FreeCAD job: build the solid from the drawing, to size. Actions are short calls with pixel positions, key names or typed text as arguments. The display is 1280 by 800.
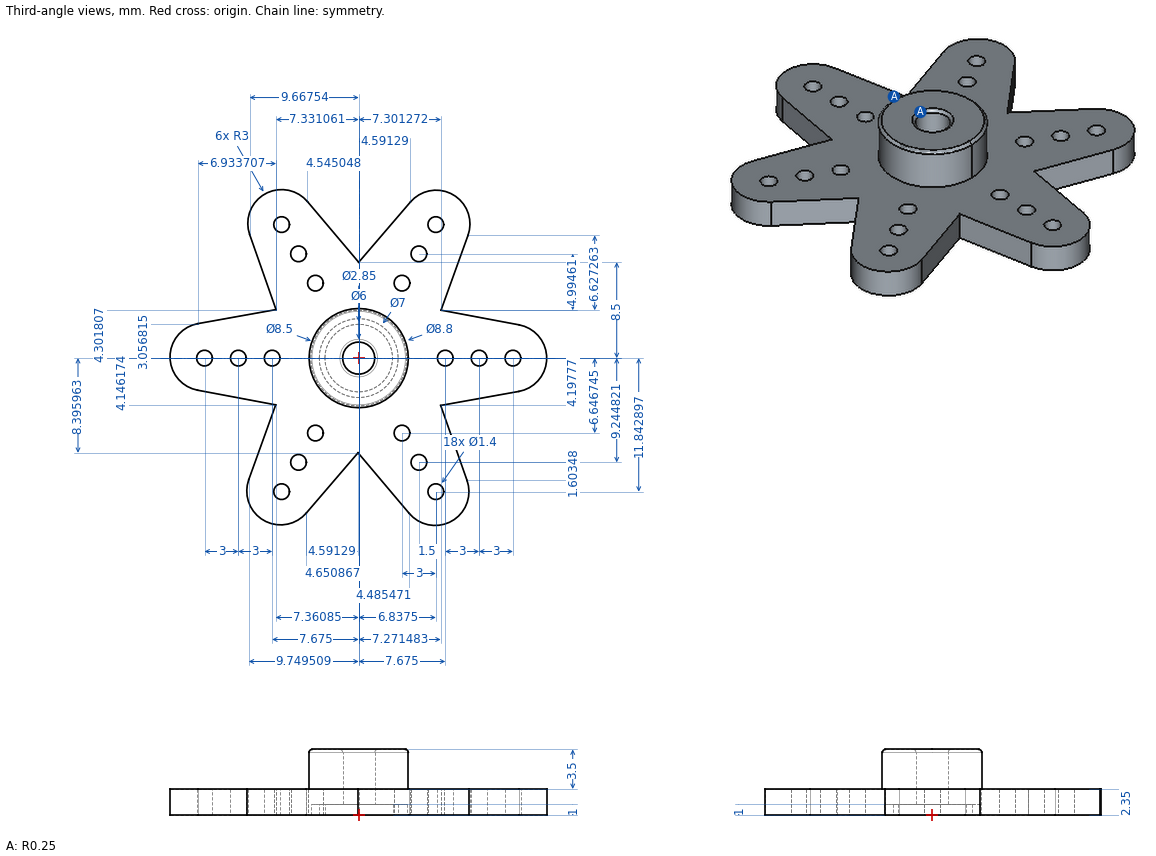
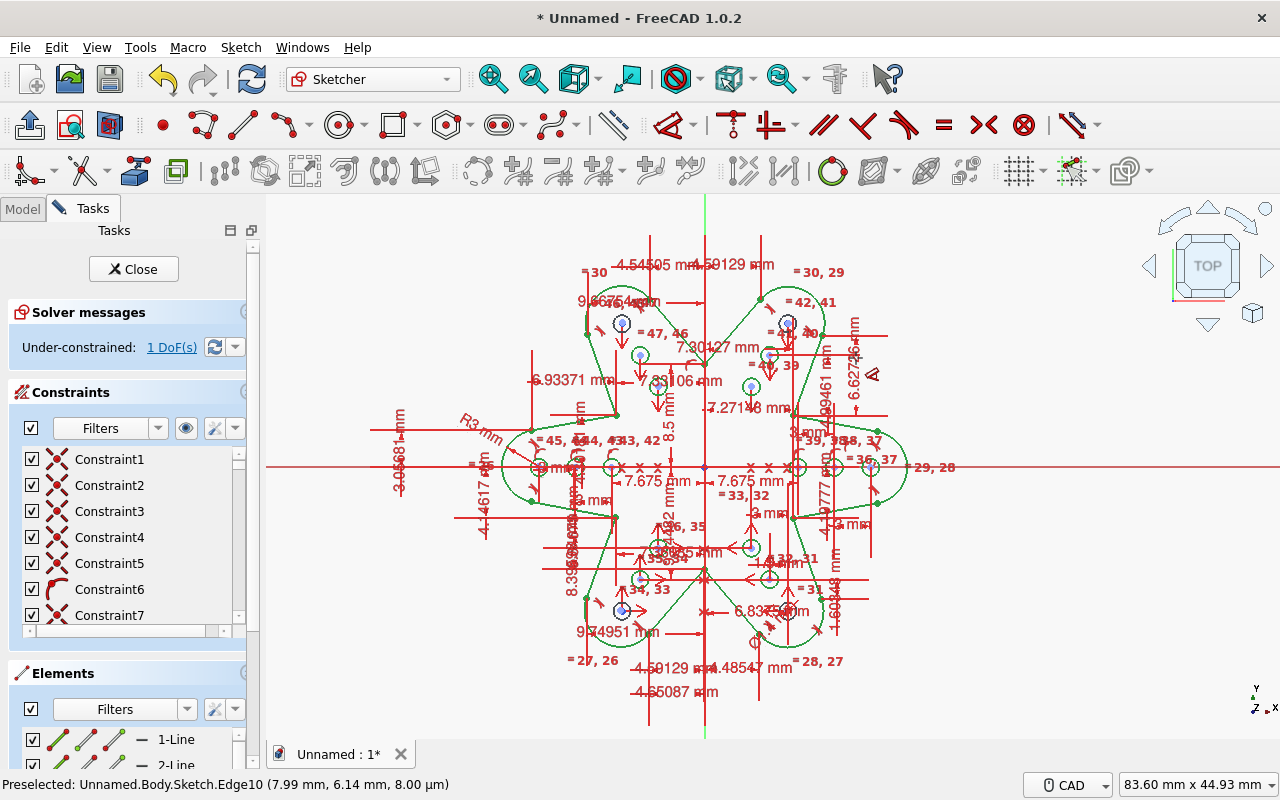
scroll(788, 611, up, 14)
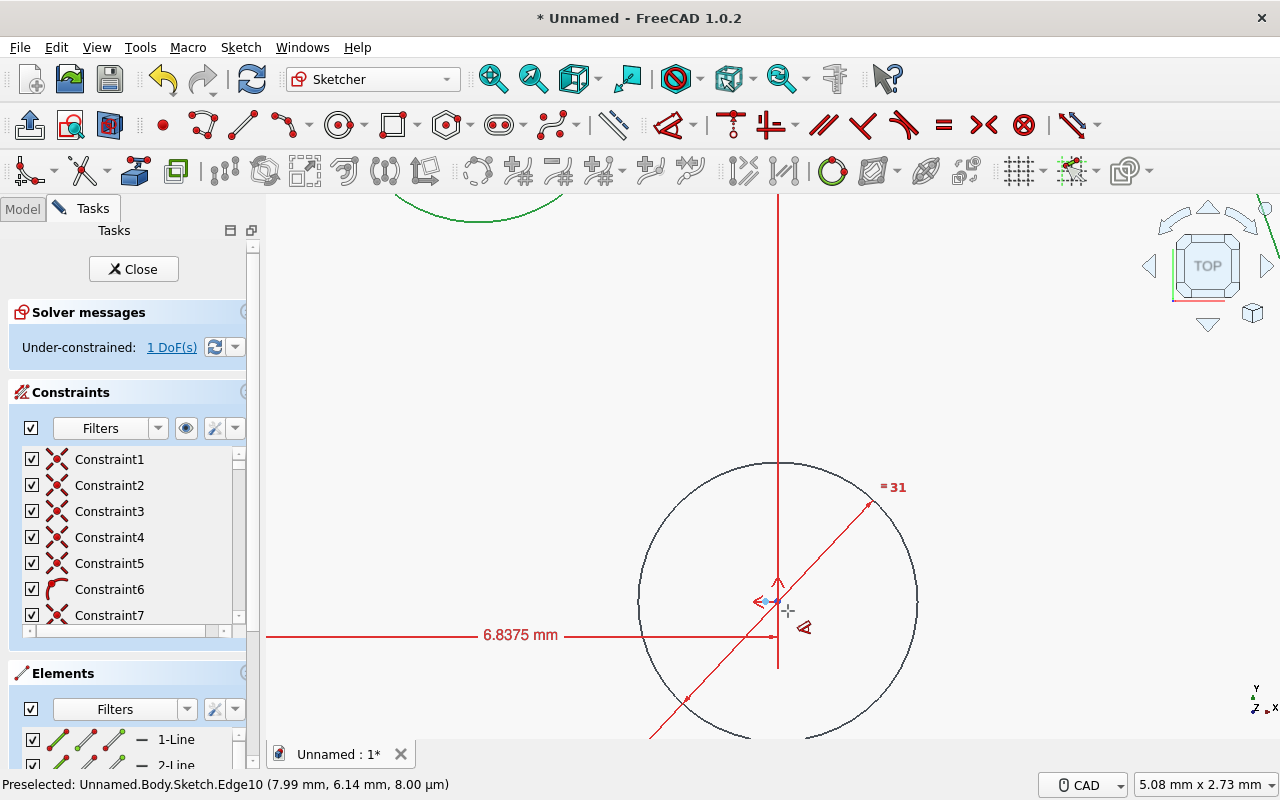
click(778, 602)
click(812, 412)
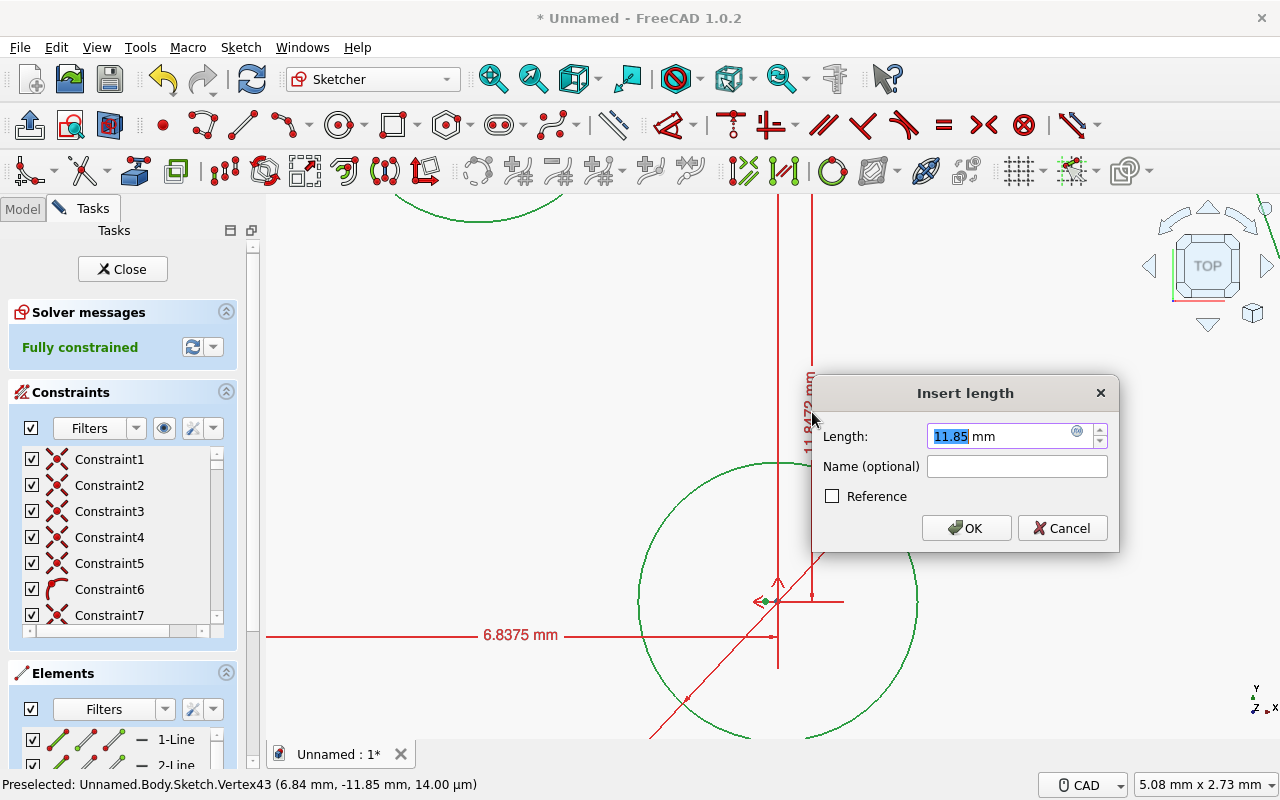
text(11.842897)
key(Return)
key(Escape)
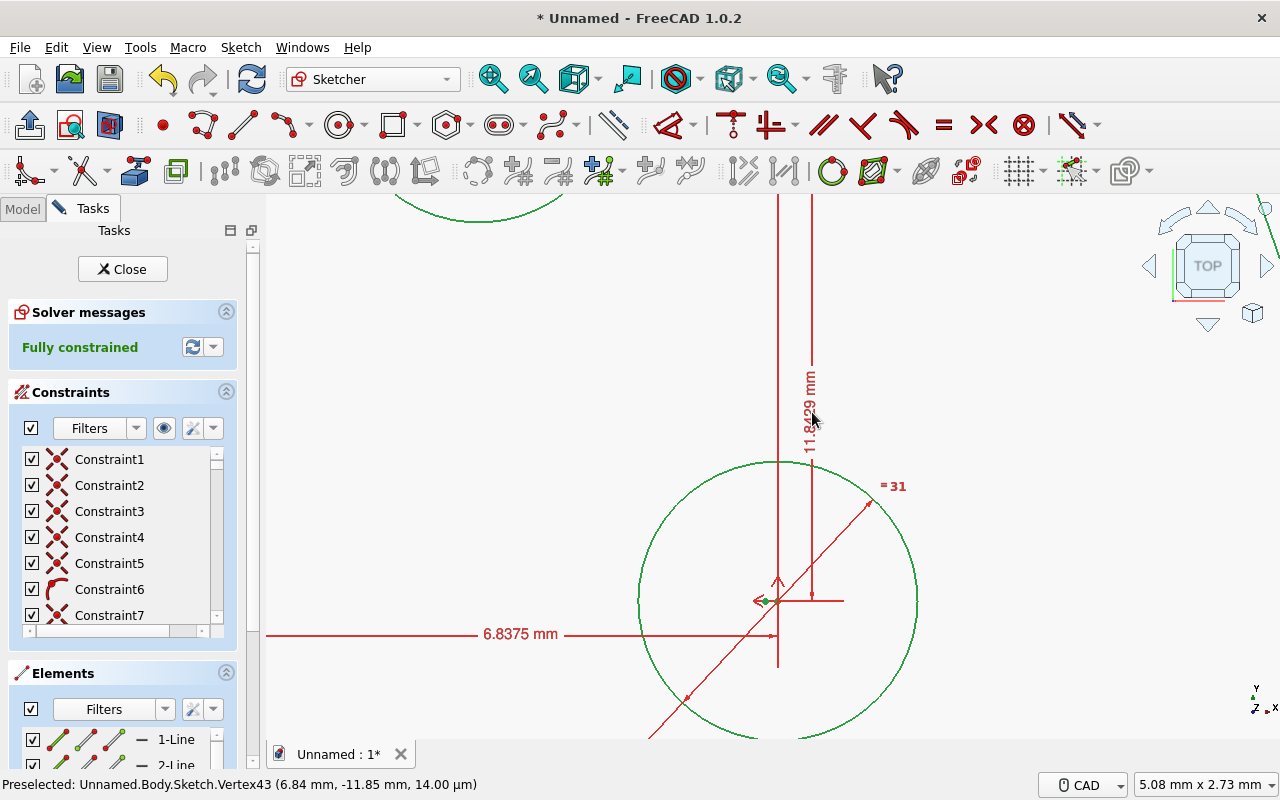
click(123, 269)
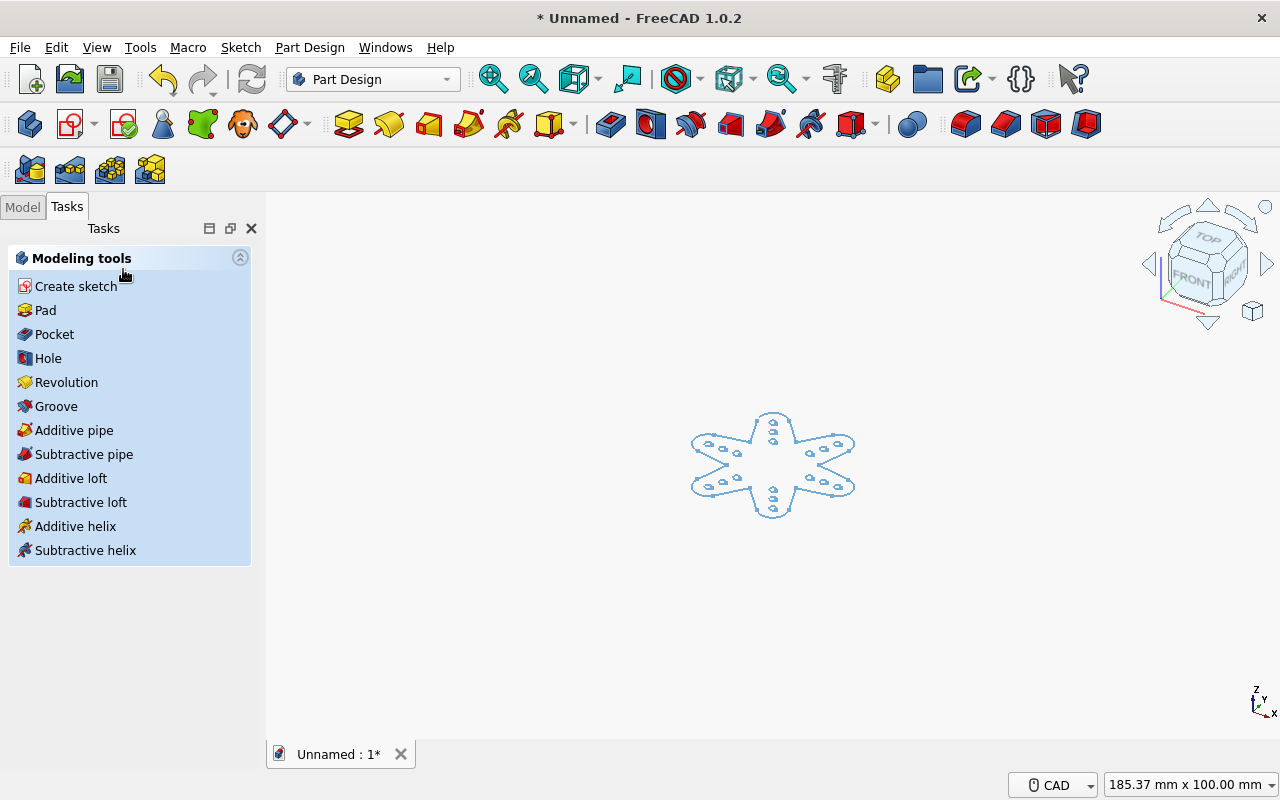
click(350, 124)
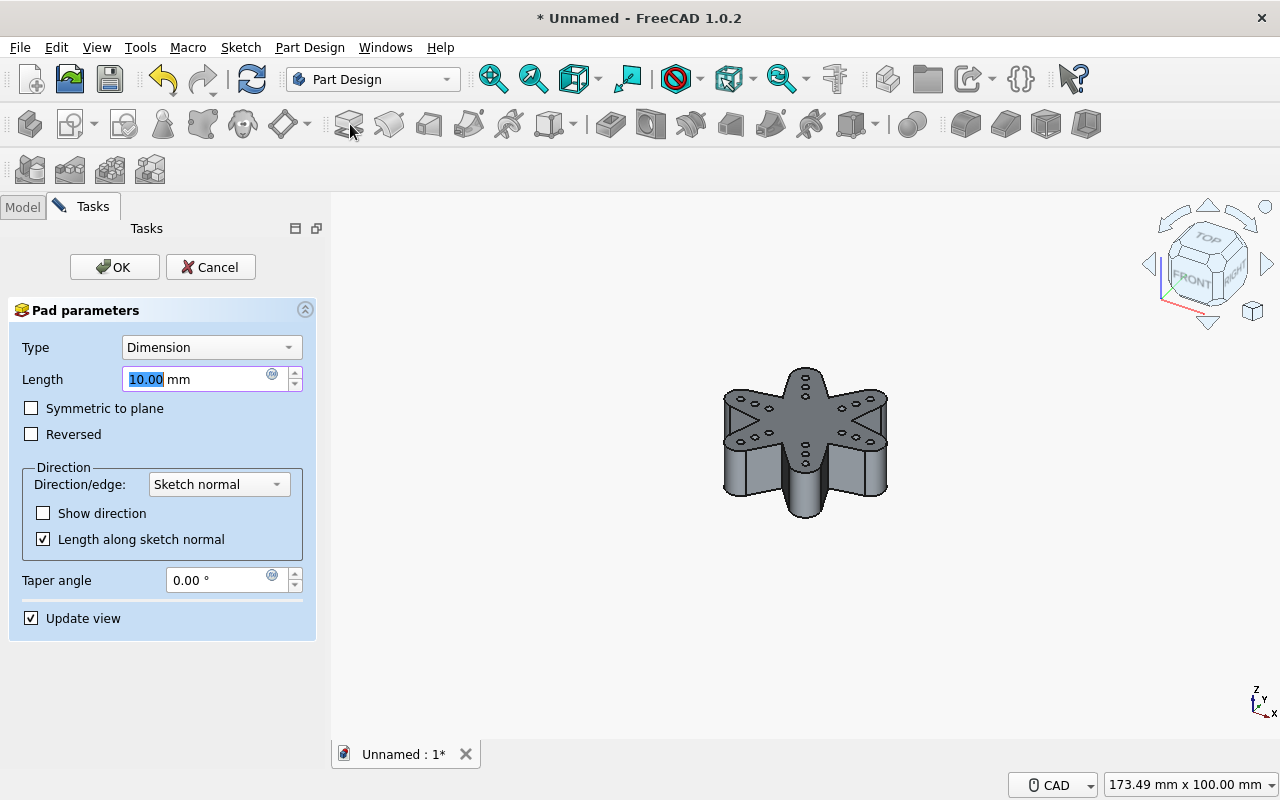
text(2.35)
key(Tab)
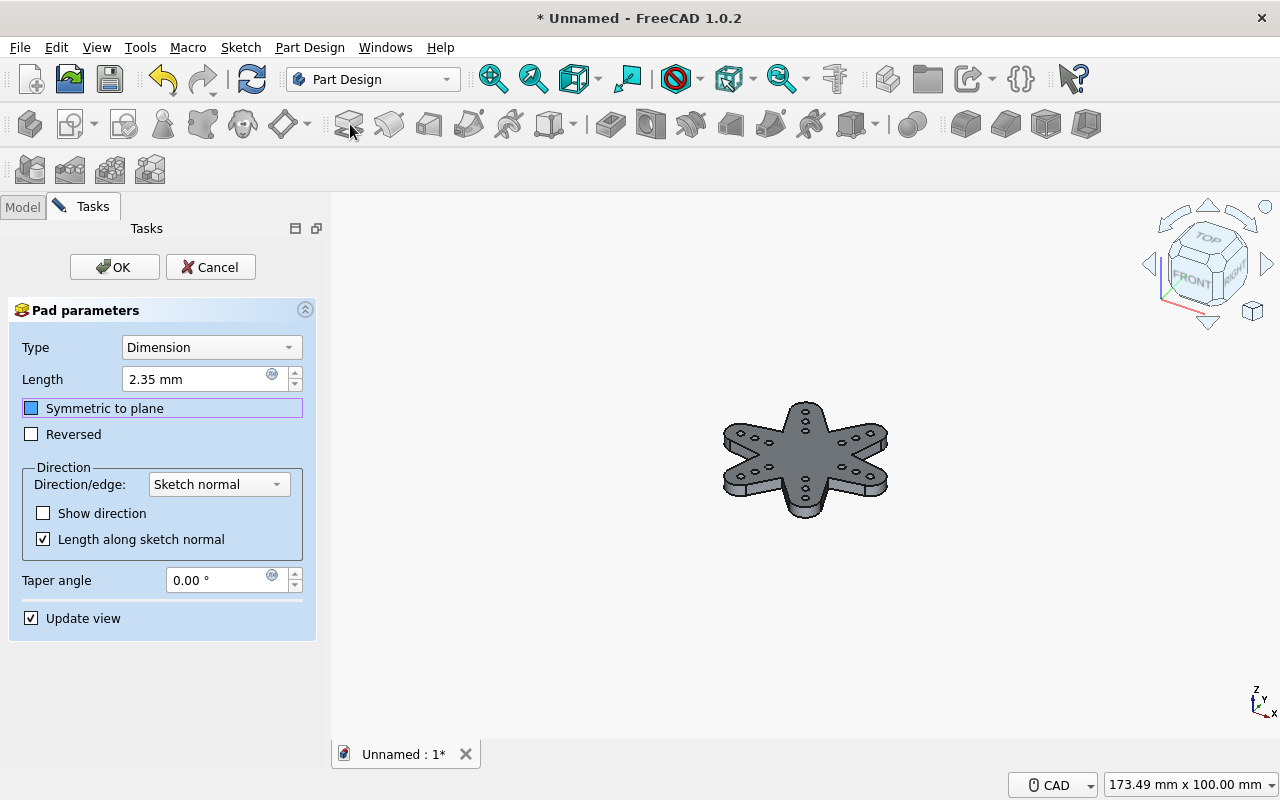
click(115, 267)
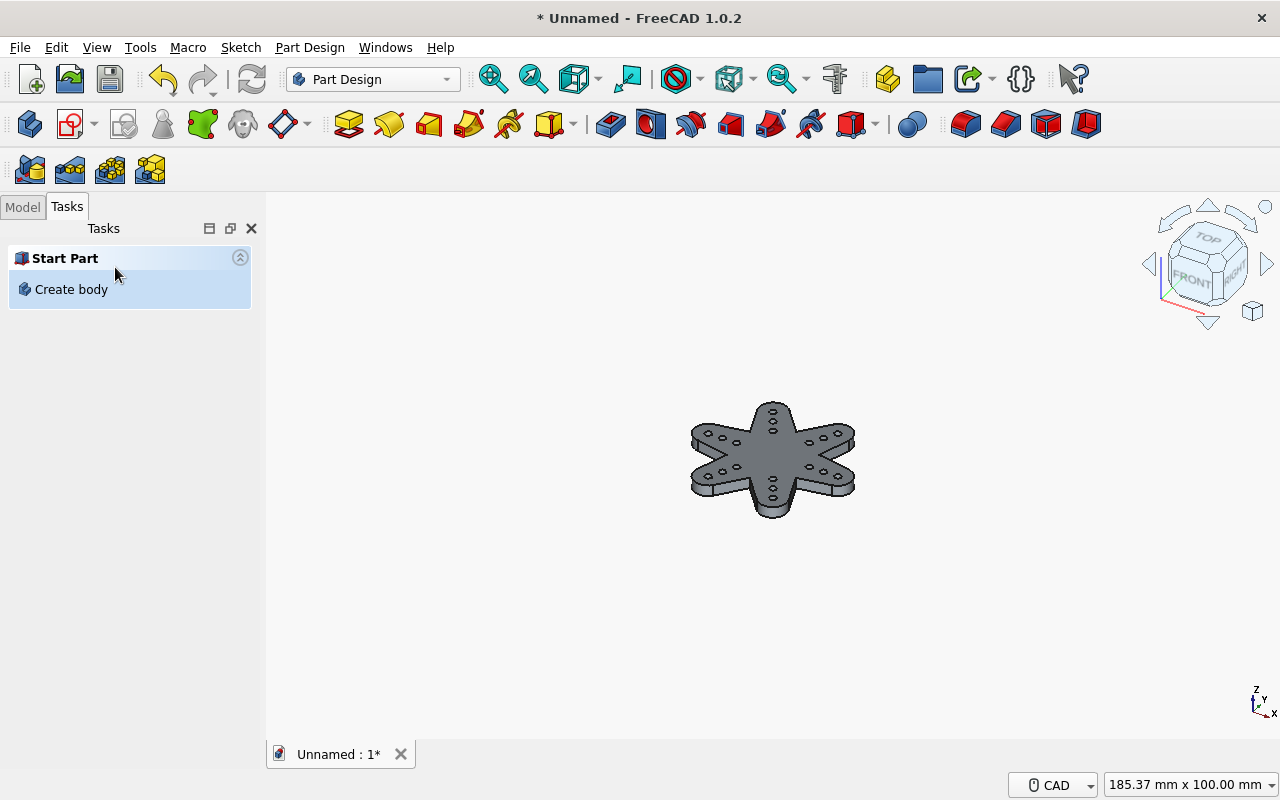
click(494, 80)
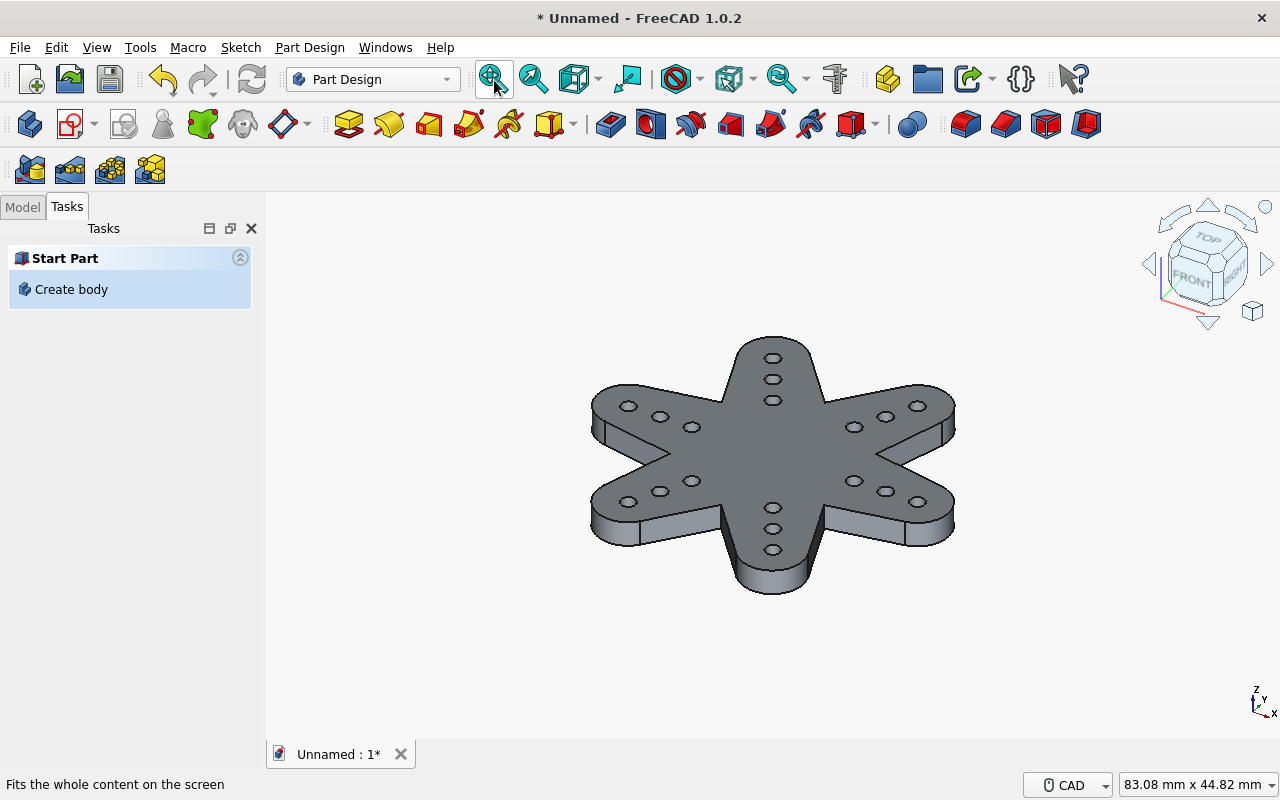
click(773, 453)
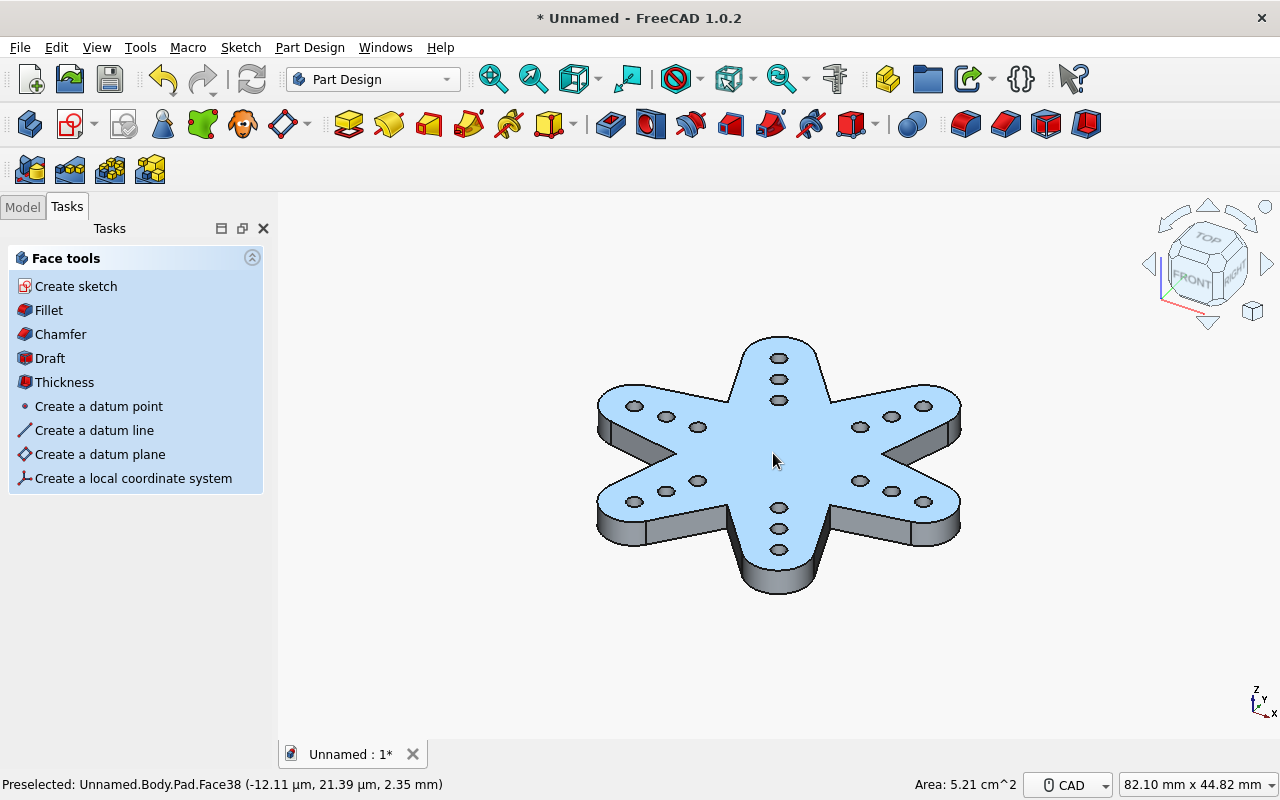
click(70, 124)